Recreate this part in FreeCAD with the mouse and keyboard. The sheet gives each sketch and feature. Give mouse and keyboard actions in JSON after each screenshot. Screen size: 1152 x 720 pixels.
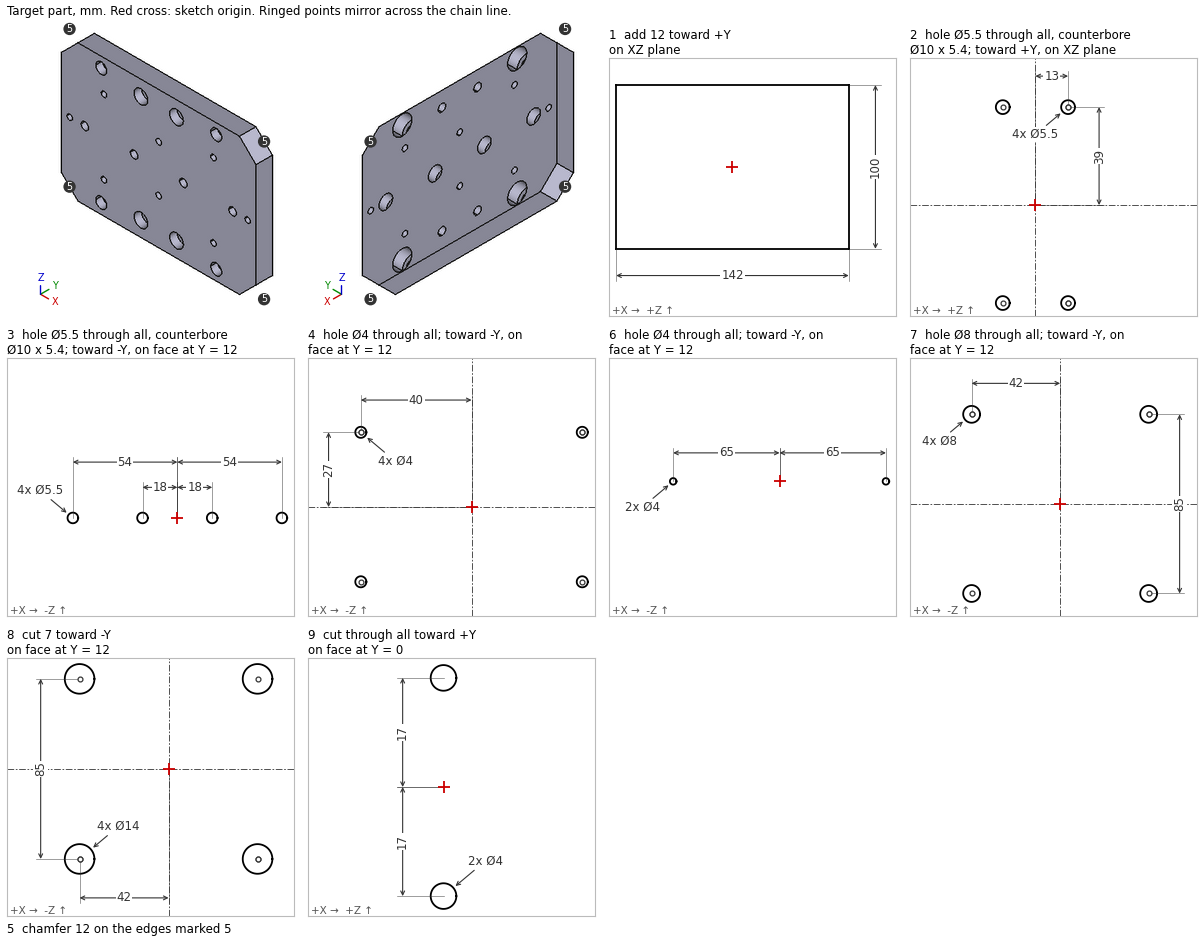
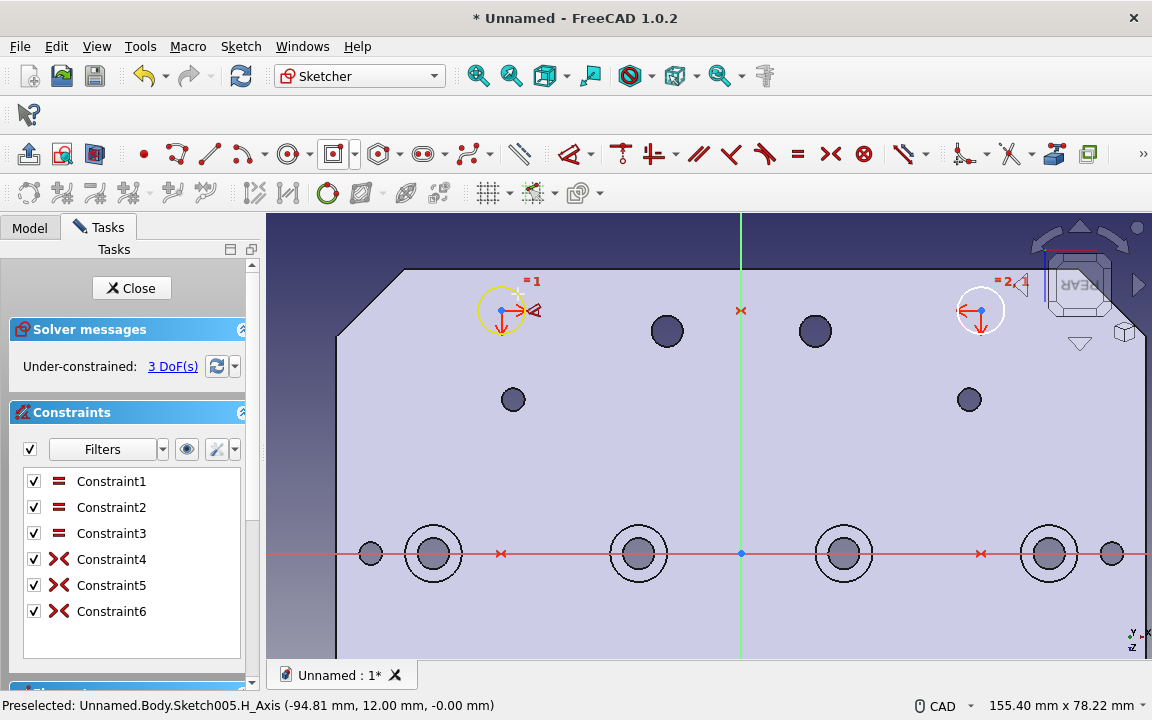
{"action": "left_click", "coordinate": [518, 294]}
{"action": "left_click", "coordinate": [541, 271]}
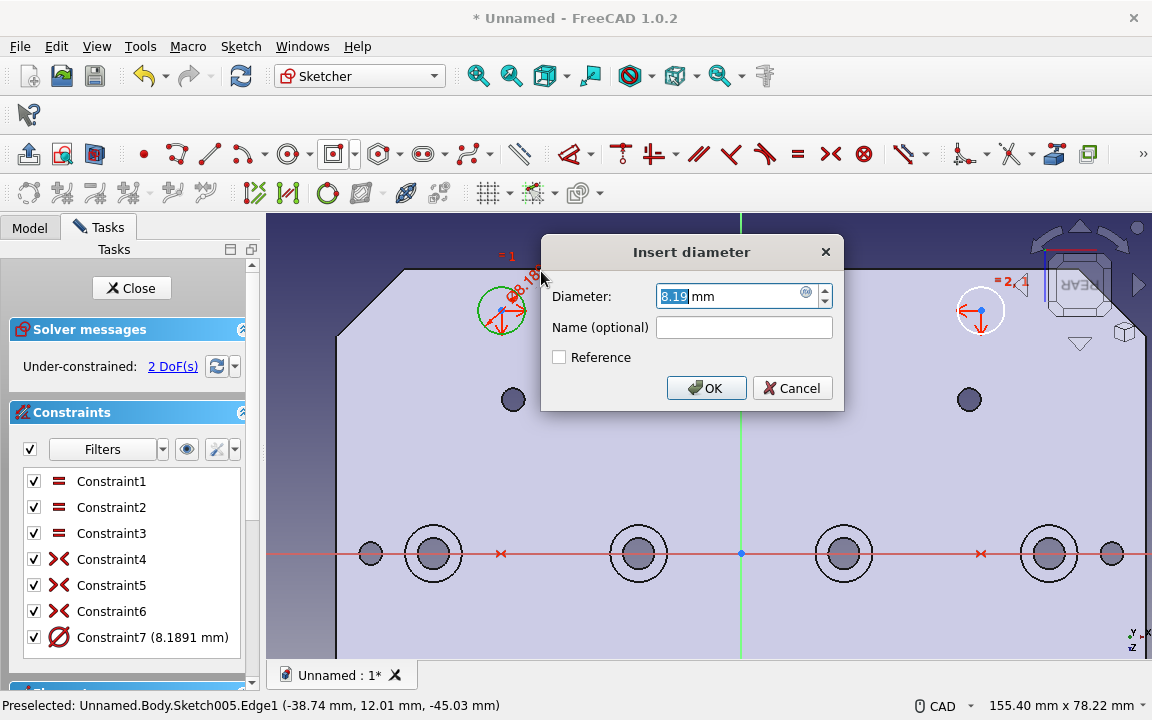
{"action": "type", "text": "8"}
{"action": "key", "text": "Return"}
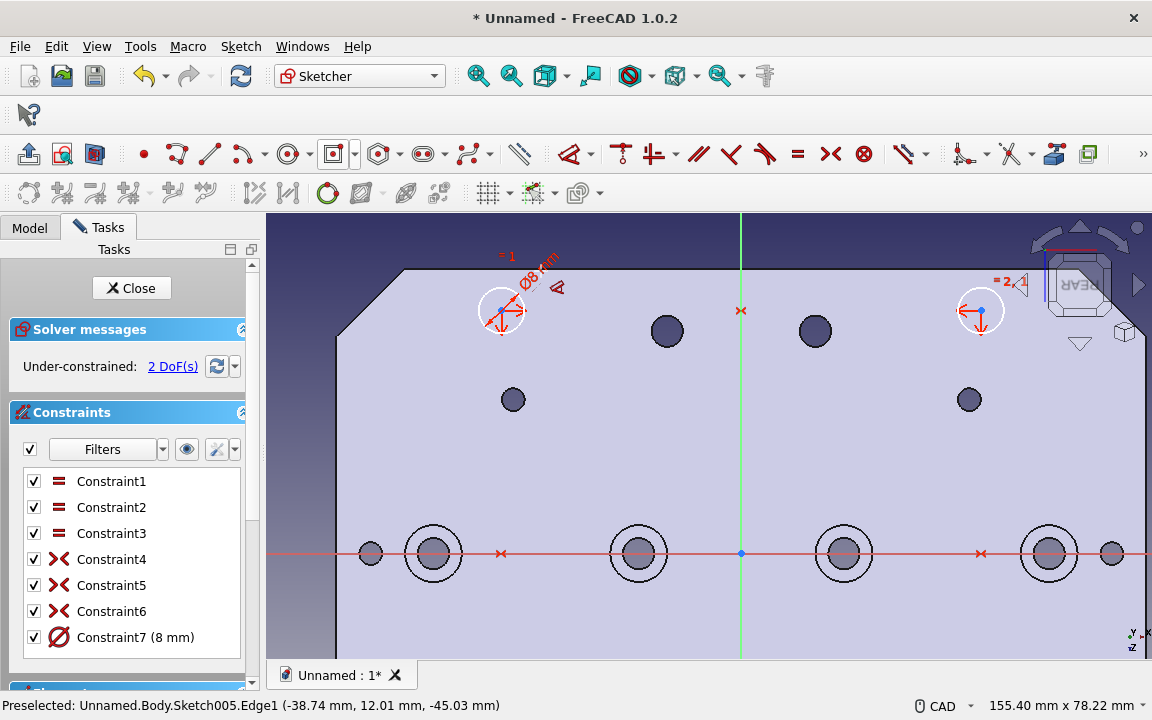
{"action": "left_click", "coordinate": [502, 311]}
{"action": "left_click", "coordinate": [621, 277]}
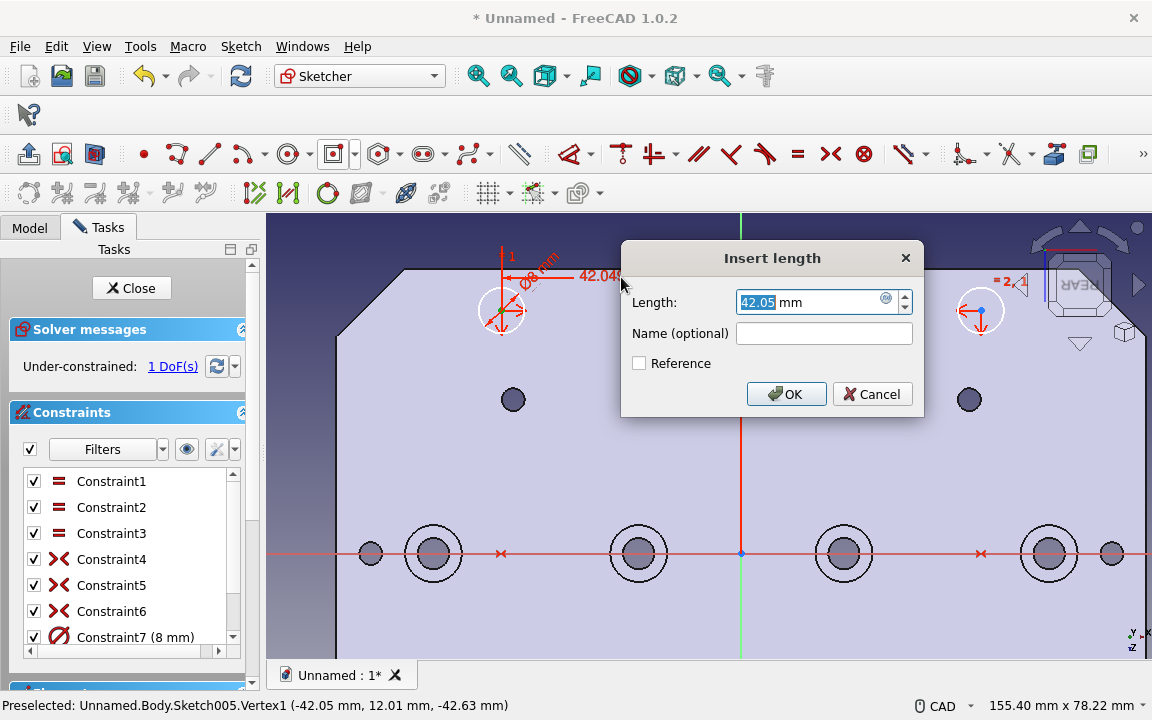
{"action": "type", "text": "42"}
{"action": "key", "text": "Return"}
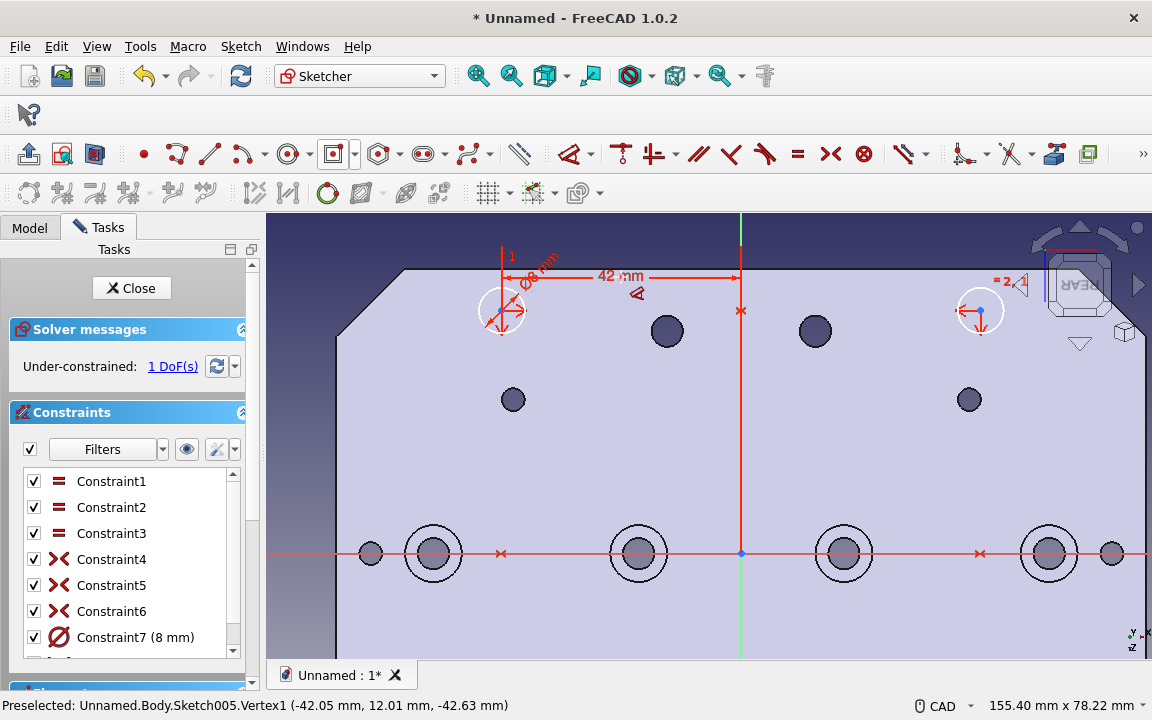
{"action": "left_click", "coordinate": [981, 311]}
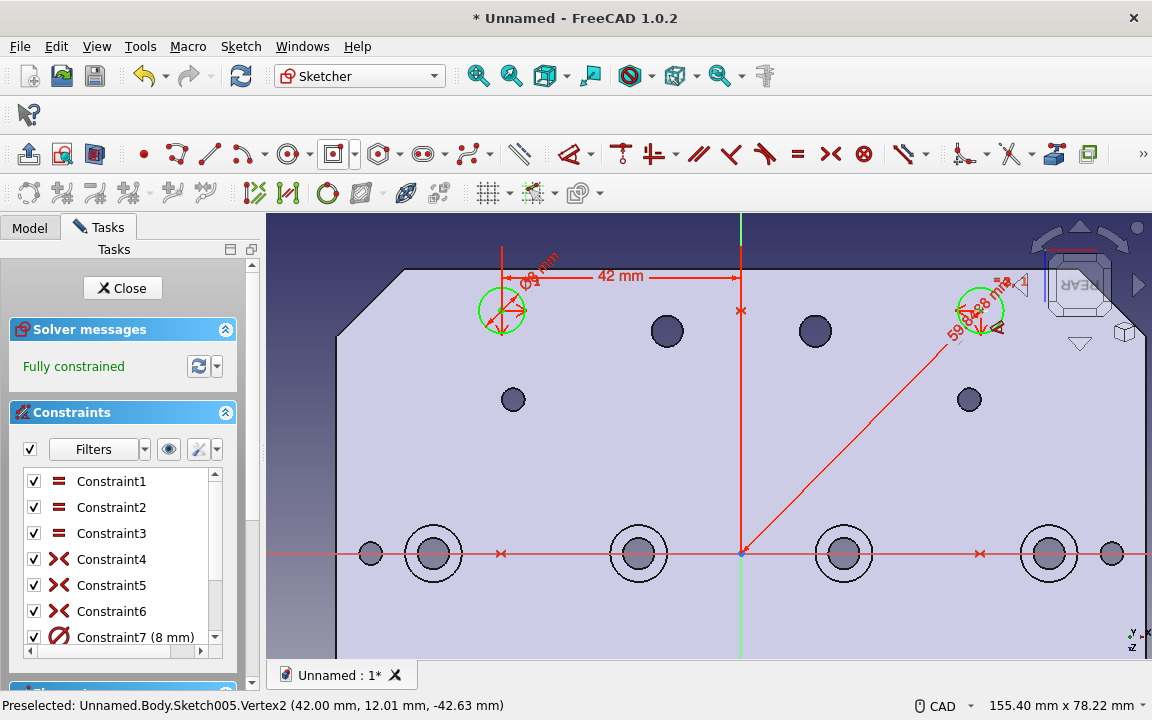
{"action": "scroll", "coordinate": [518, 293], "scroll_direction": "down", "scroll_amount": 3}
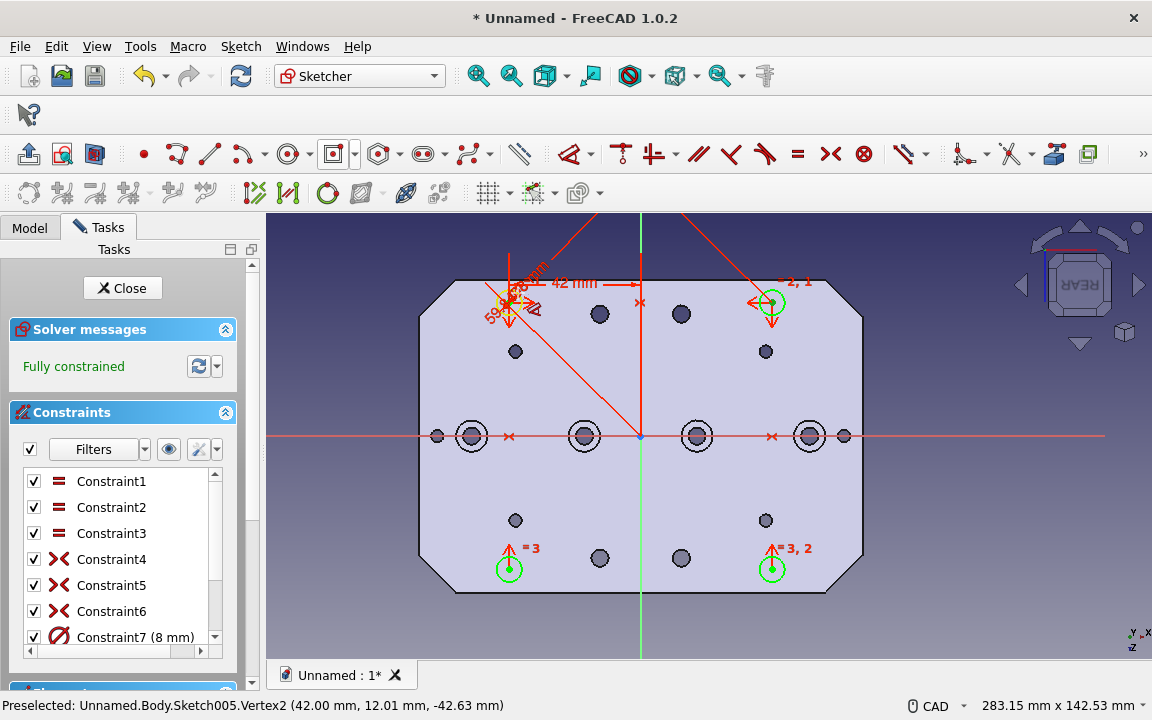
{"action": "left_click", "coordinate": [772, 569]}
{"action": "left_click", "coordinate": [806, 375]}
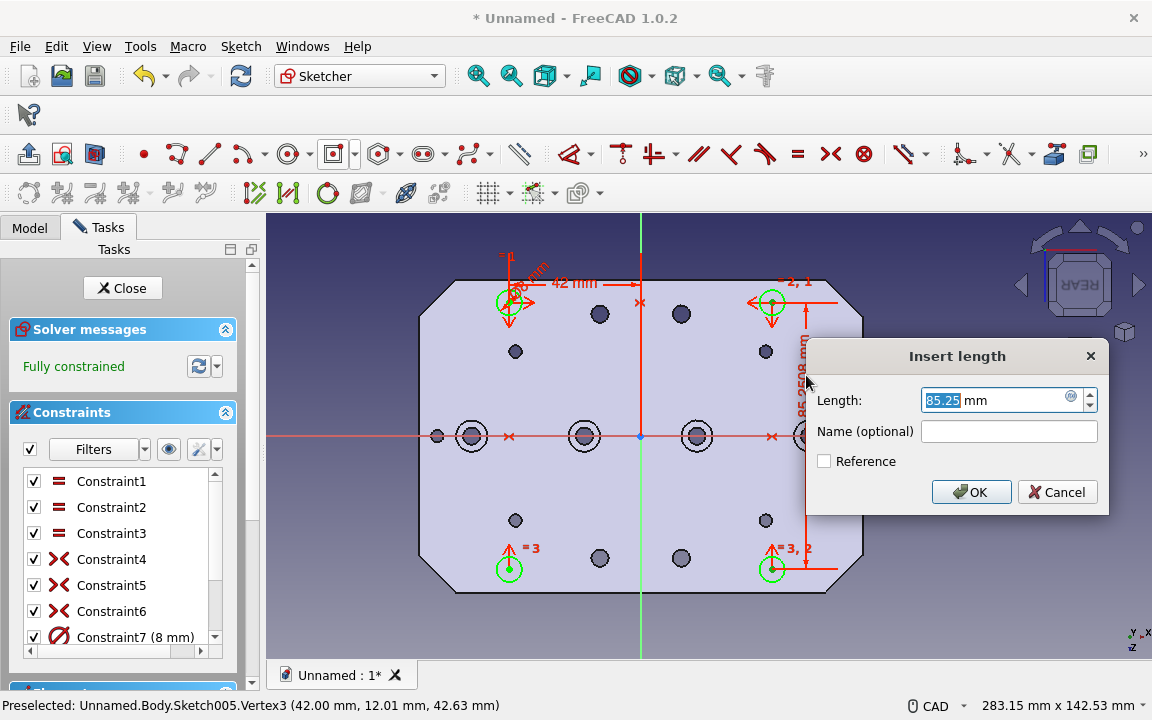
{"action": "type", "text": "85"}
{"action": "key", "text": "Return"}
{"action": "key", "text": "Escape"}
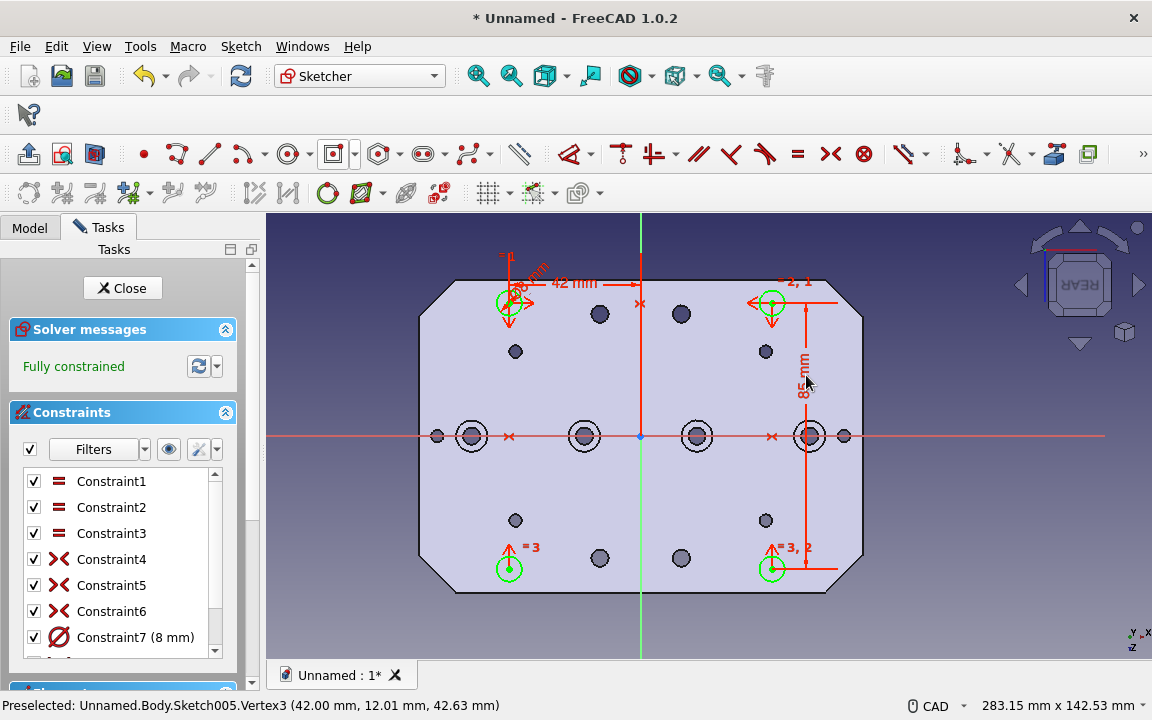
{"action": "left_click", "coordinate": [123, 288]}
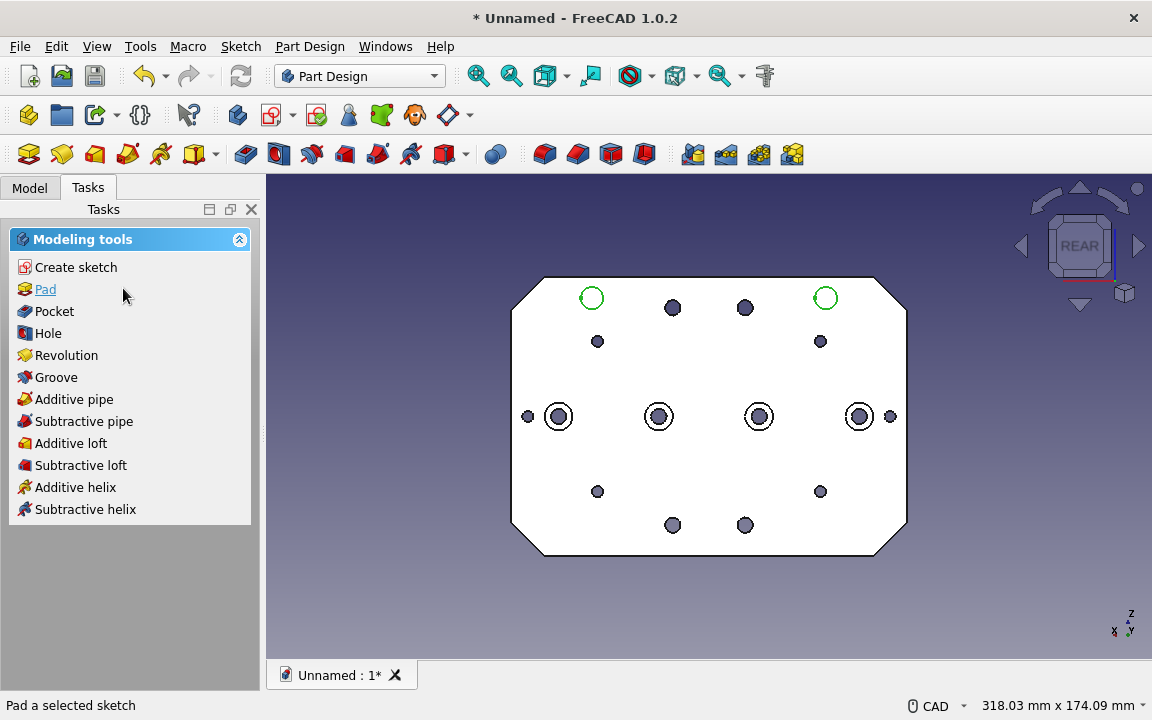
{"action": "left_click", "coordinate": [279, 154]}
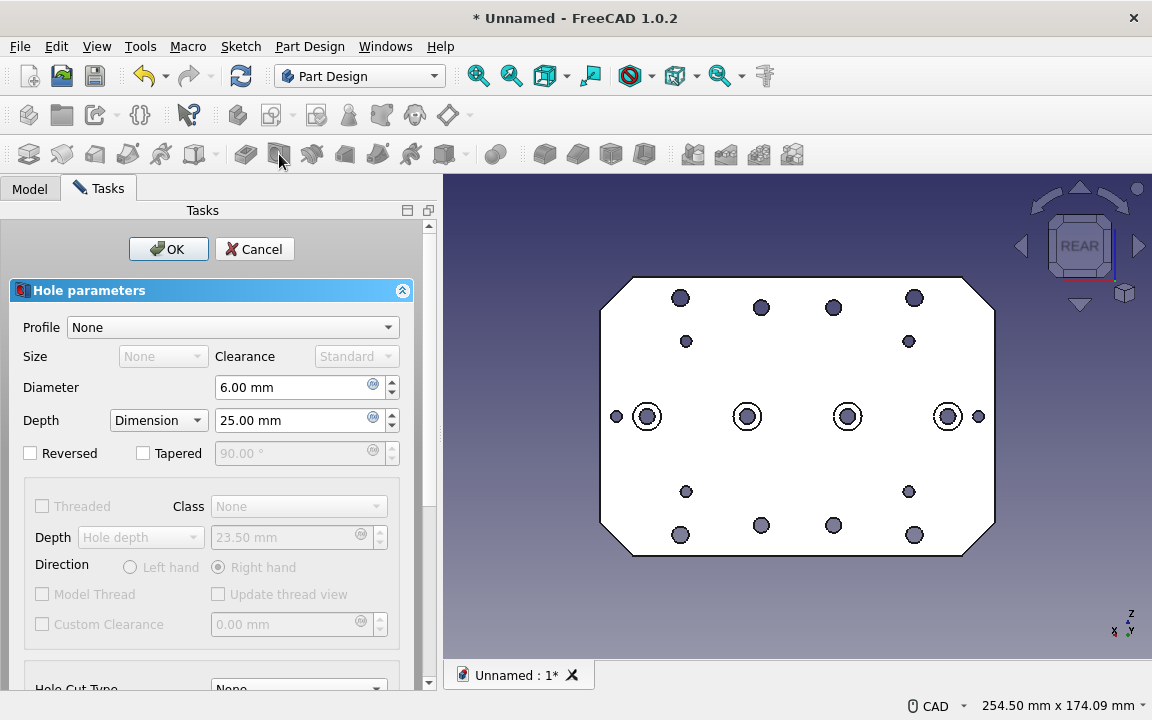
{"action": "triple_click", "coordinate": [300, 388]}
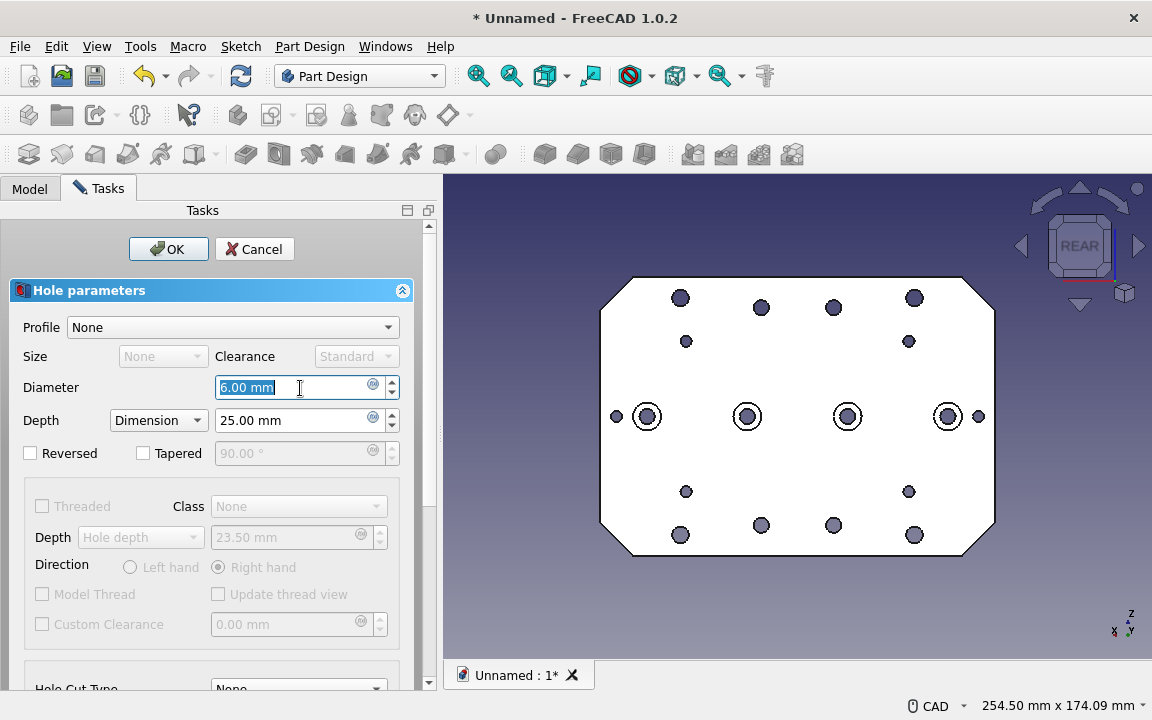
{"action": "type", "text": "8"}
{"action": "key", "text": "Tab"}